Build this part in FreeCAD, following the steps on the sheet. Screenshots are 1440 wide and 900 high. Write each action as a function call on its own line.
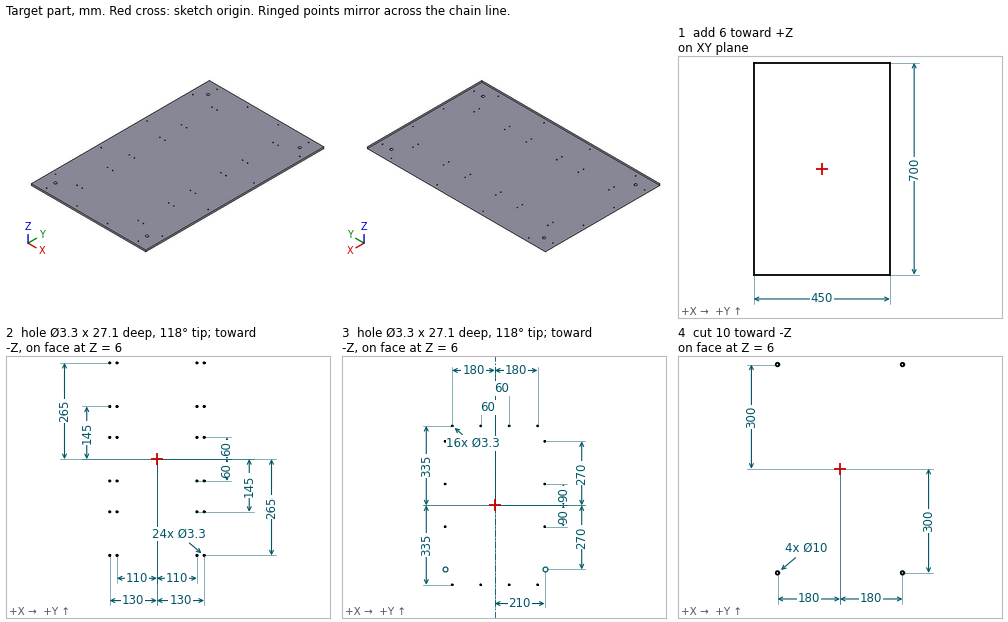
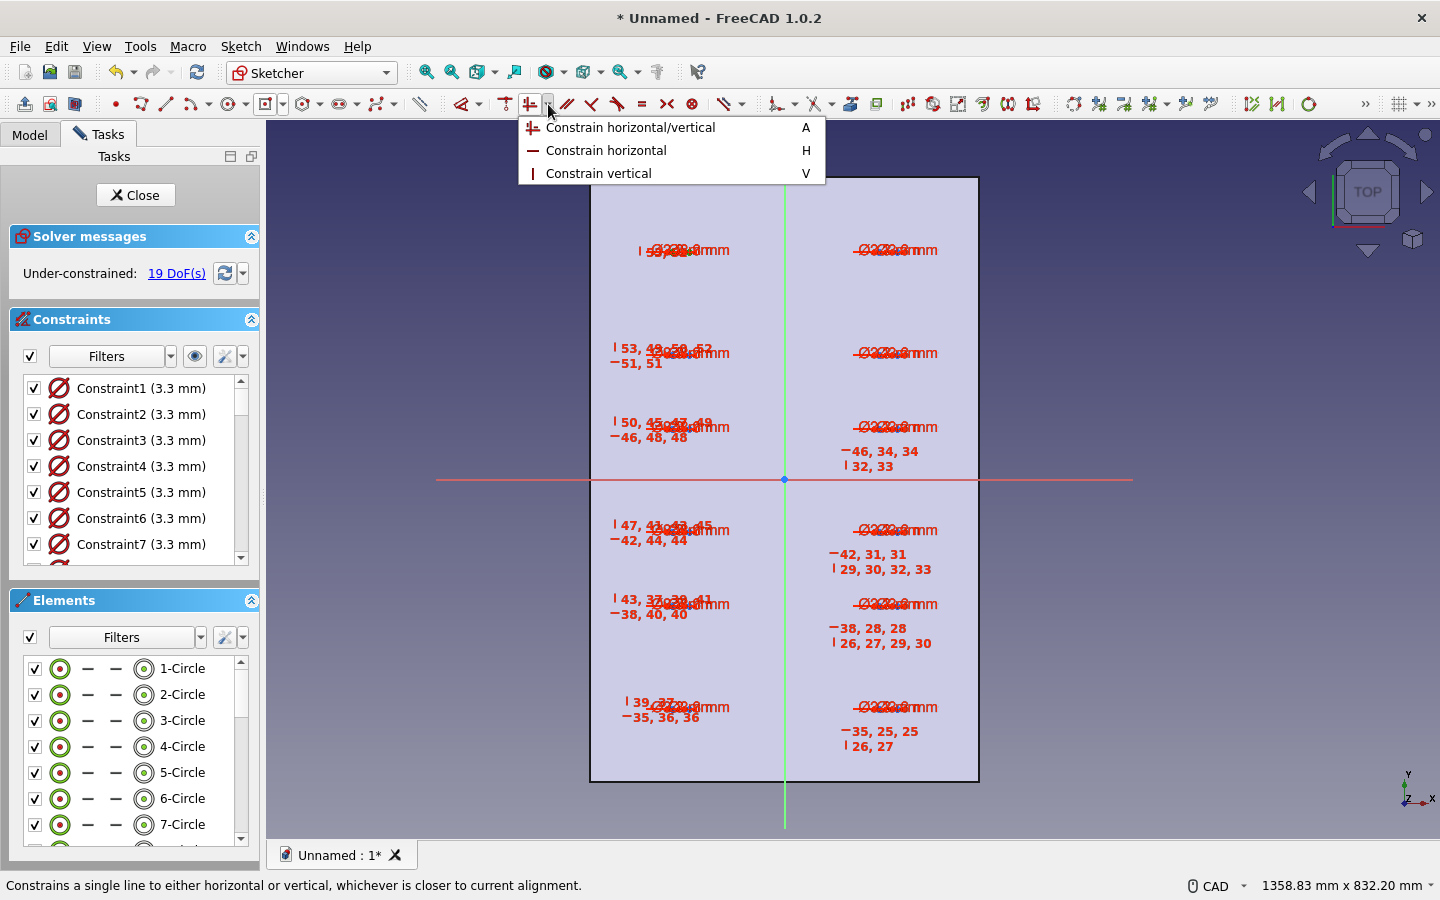
click(672, 150)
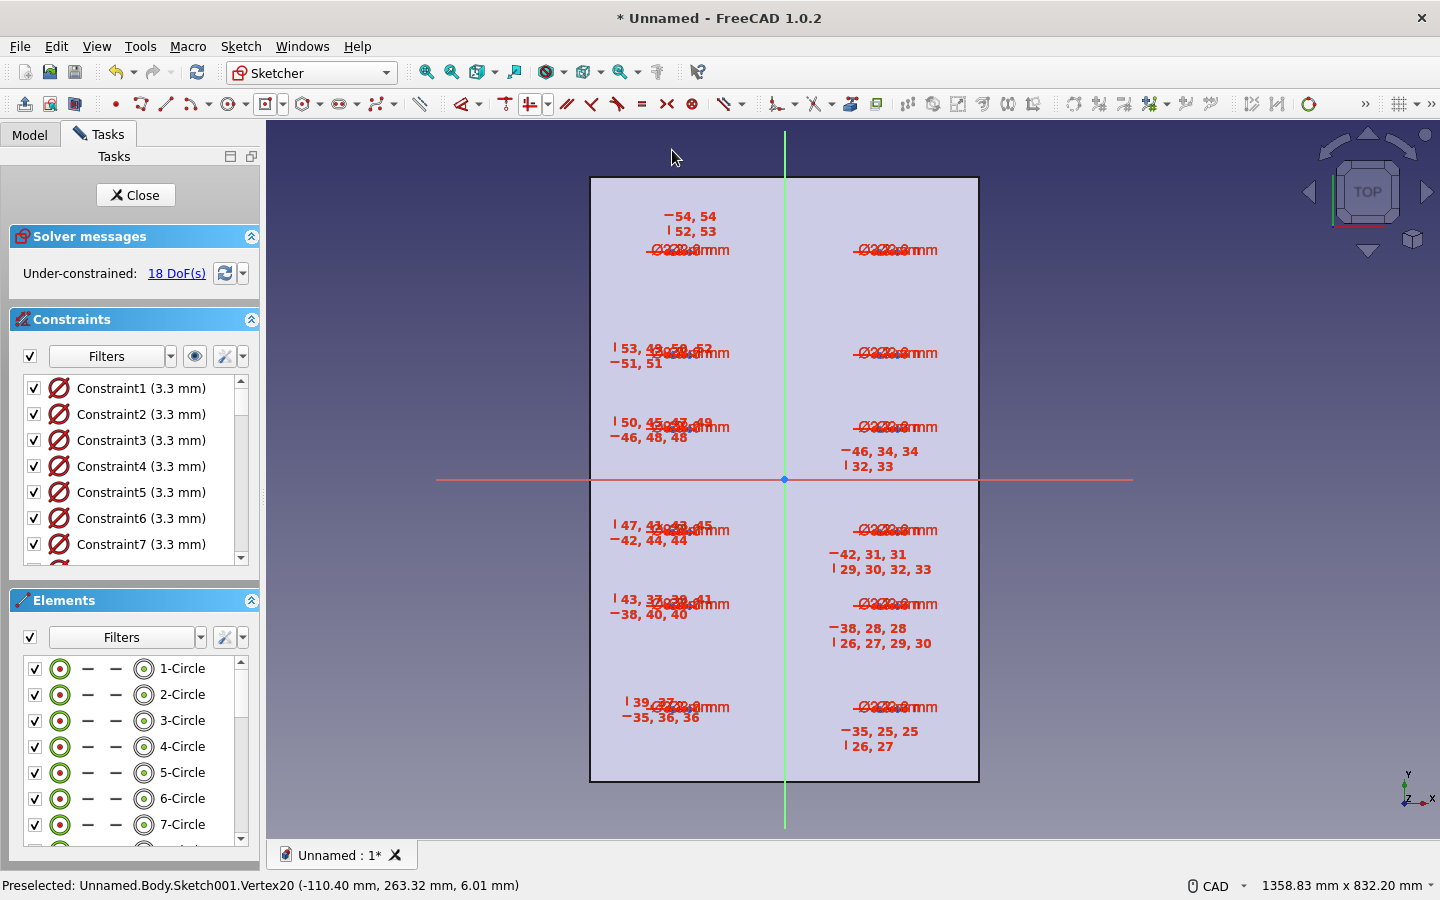
click(879, 429)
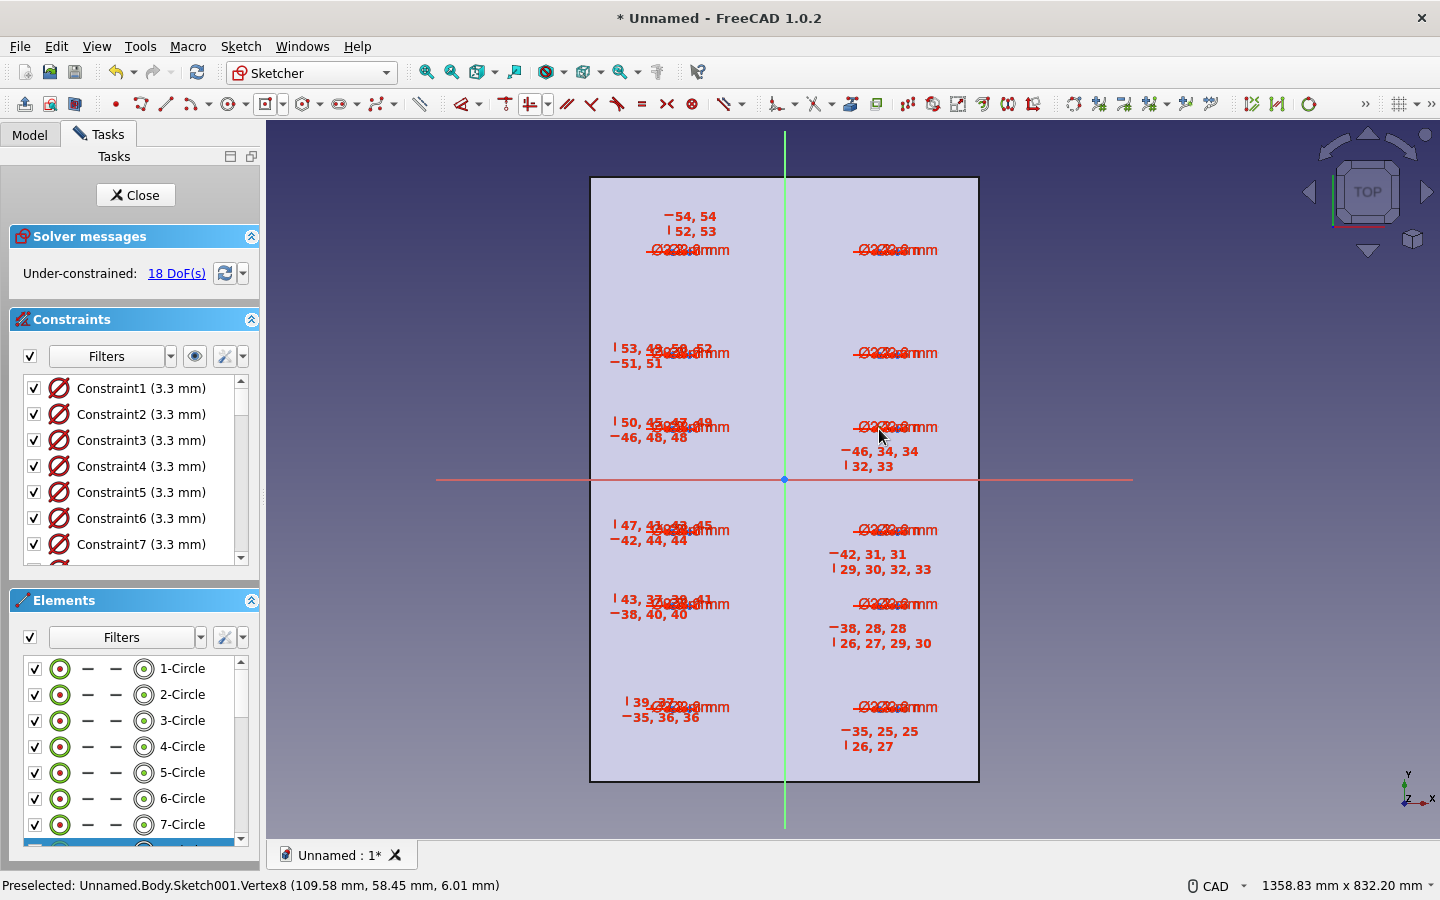
click(879, 355)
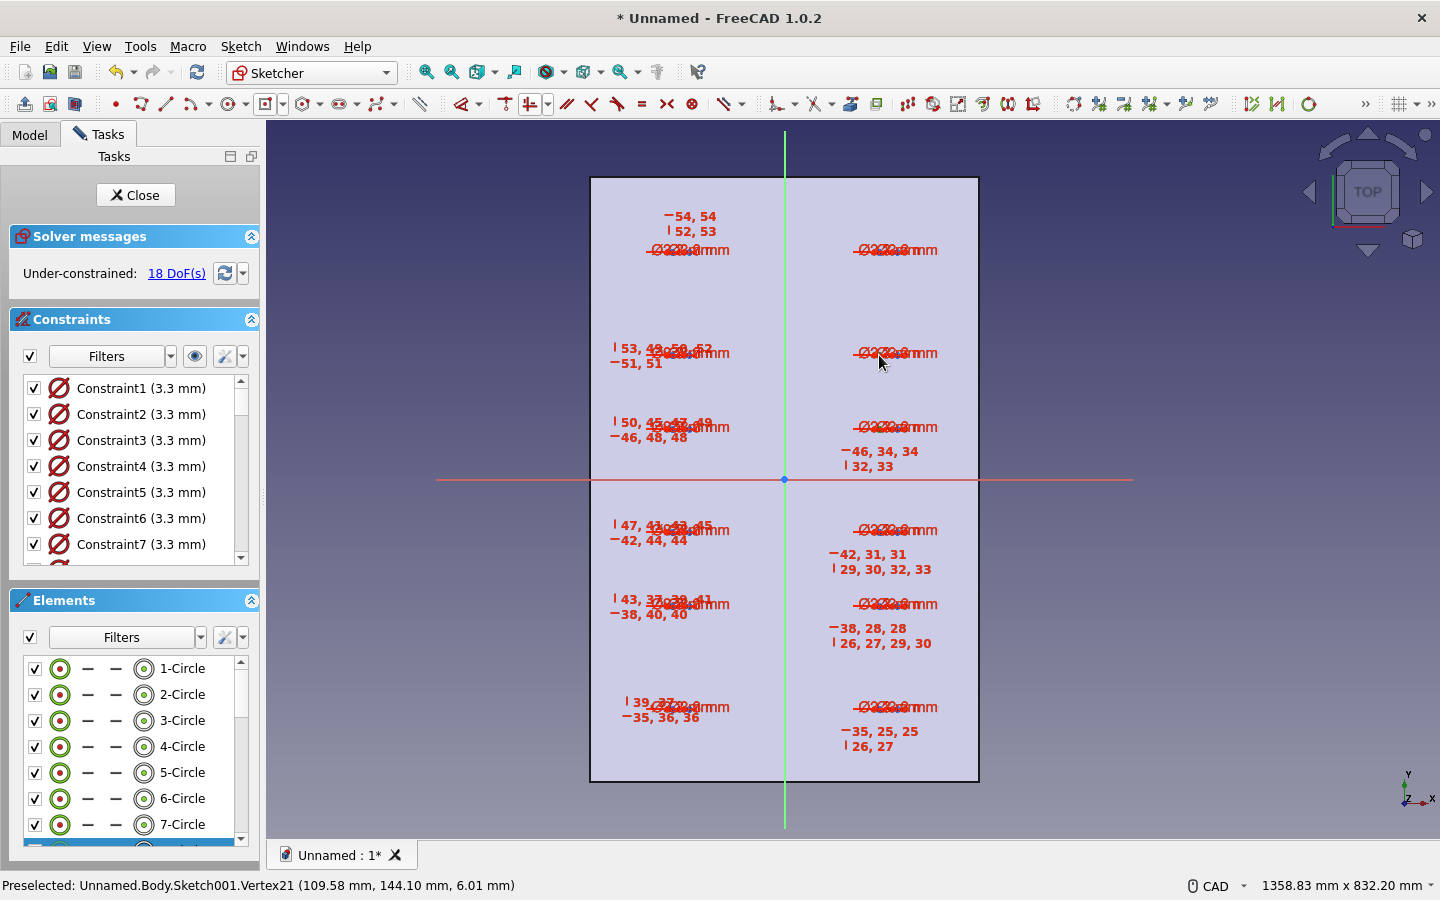
key(v)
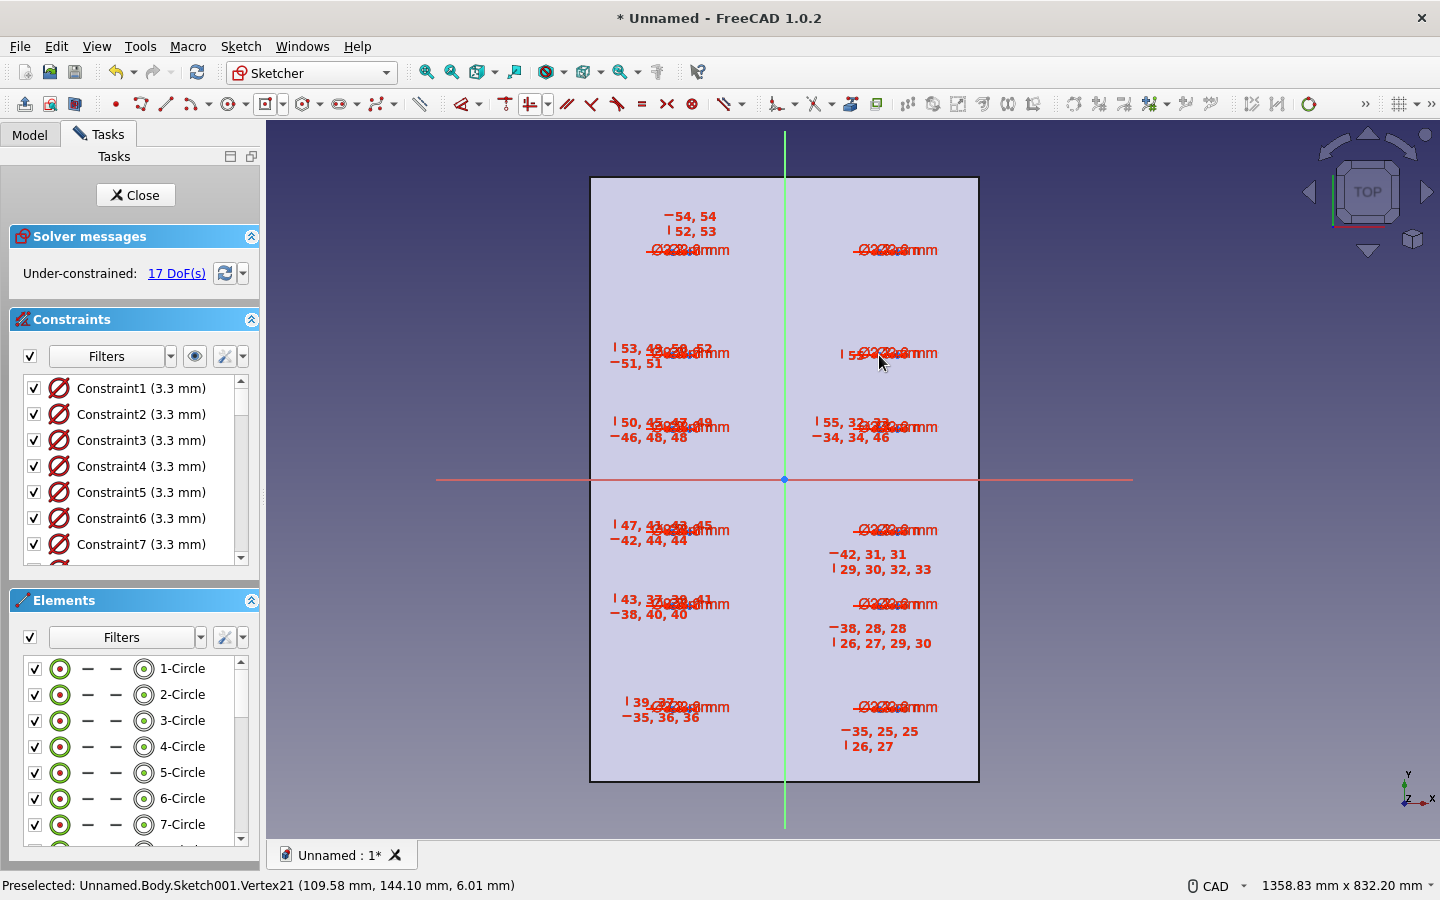
click(689, 355)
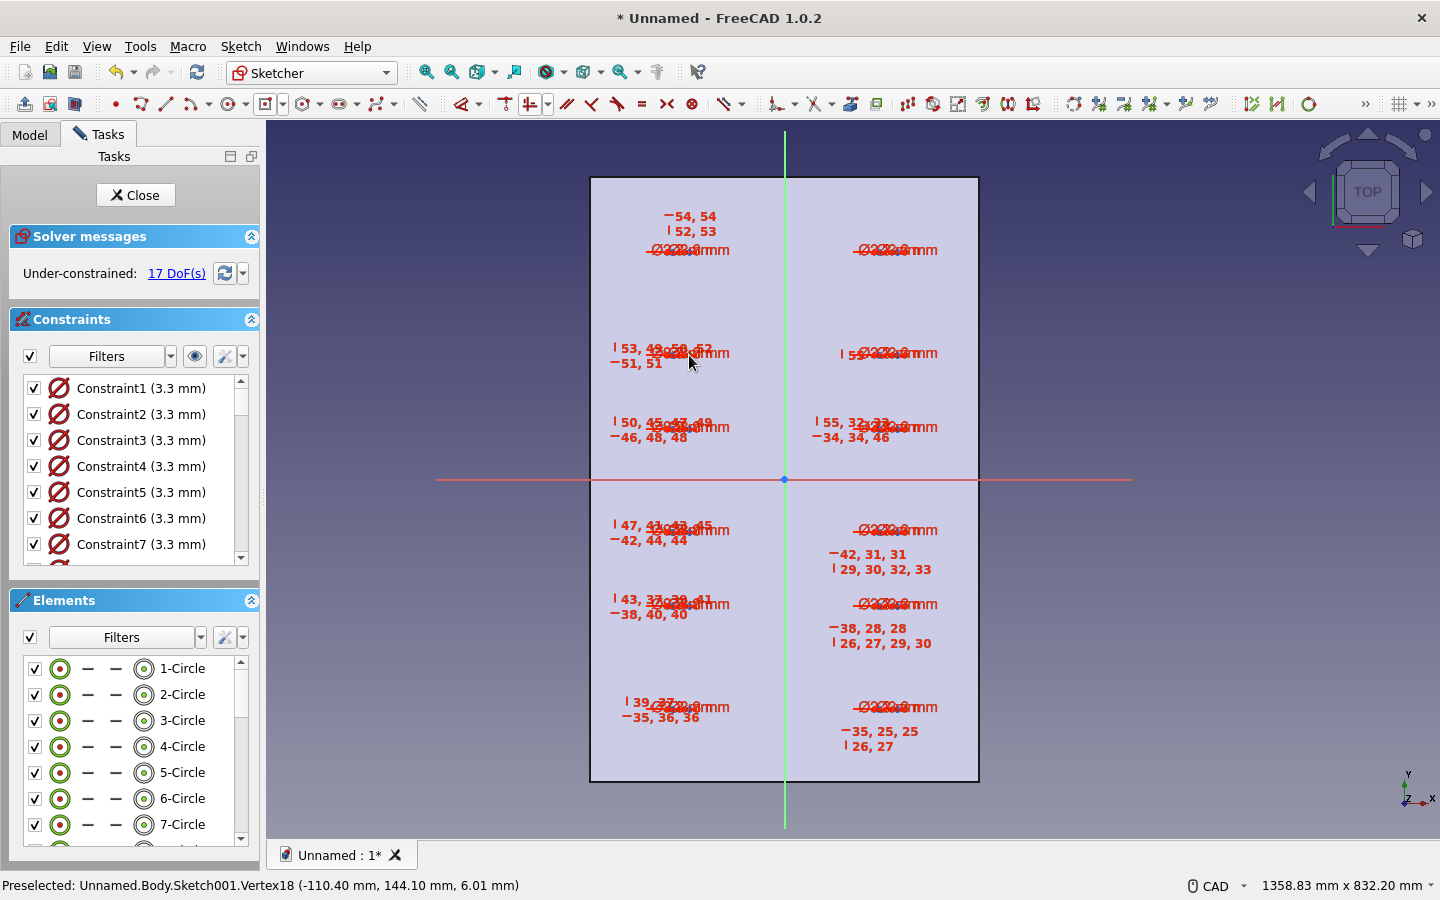
click(879, 355)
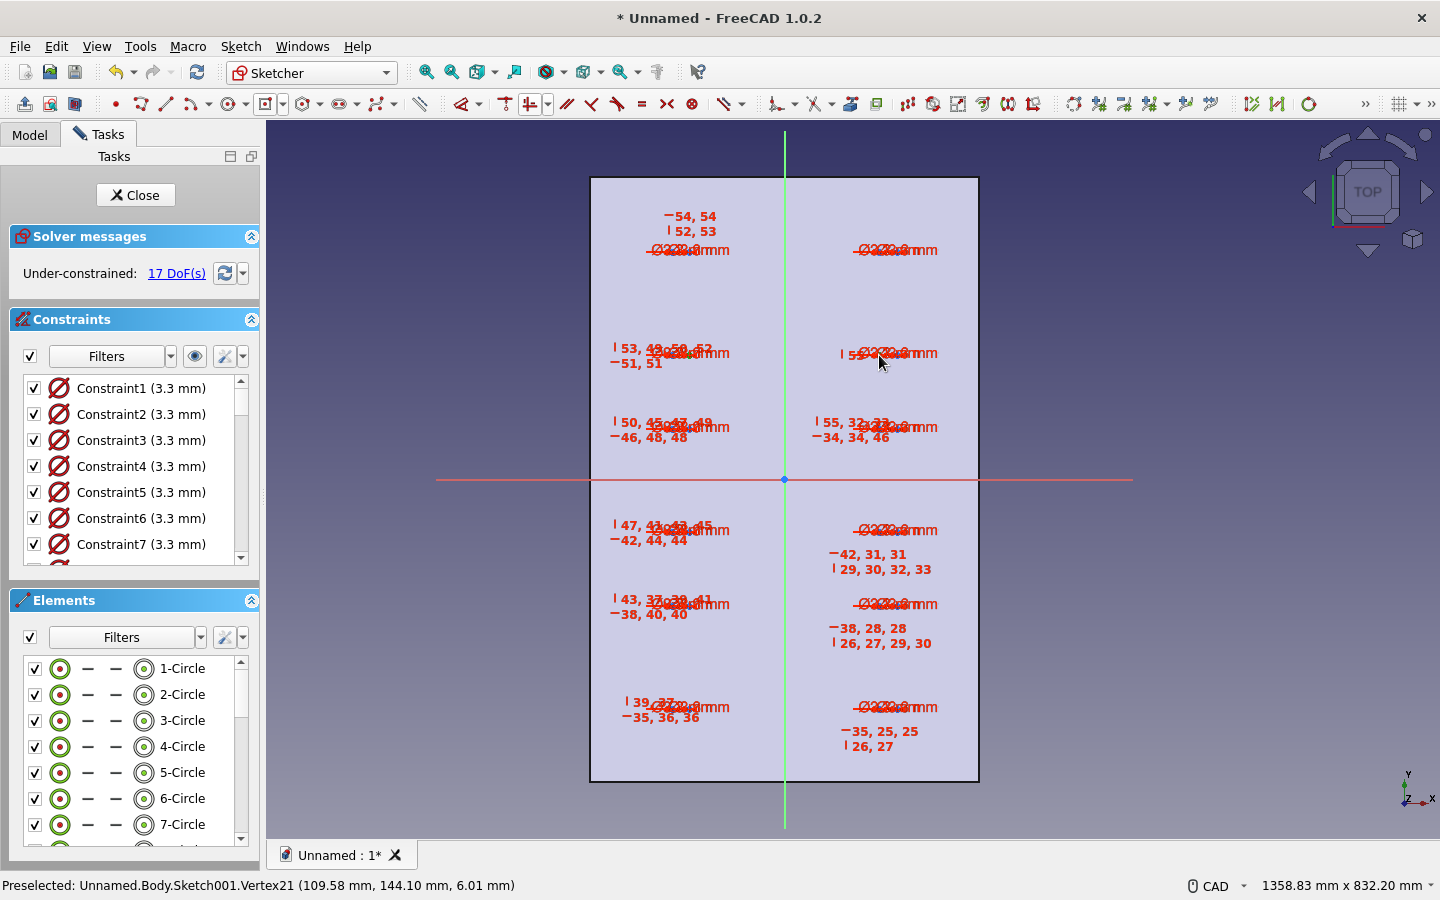
click(548, 104)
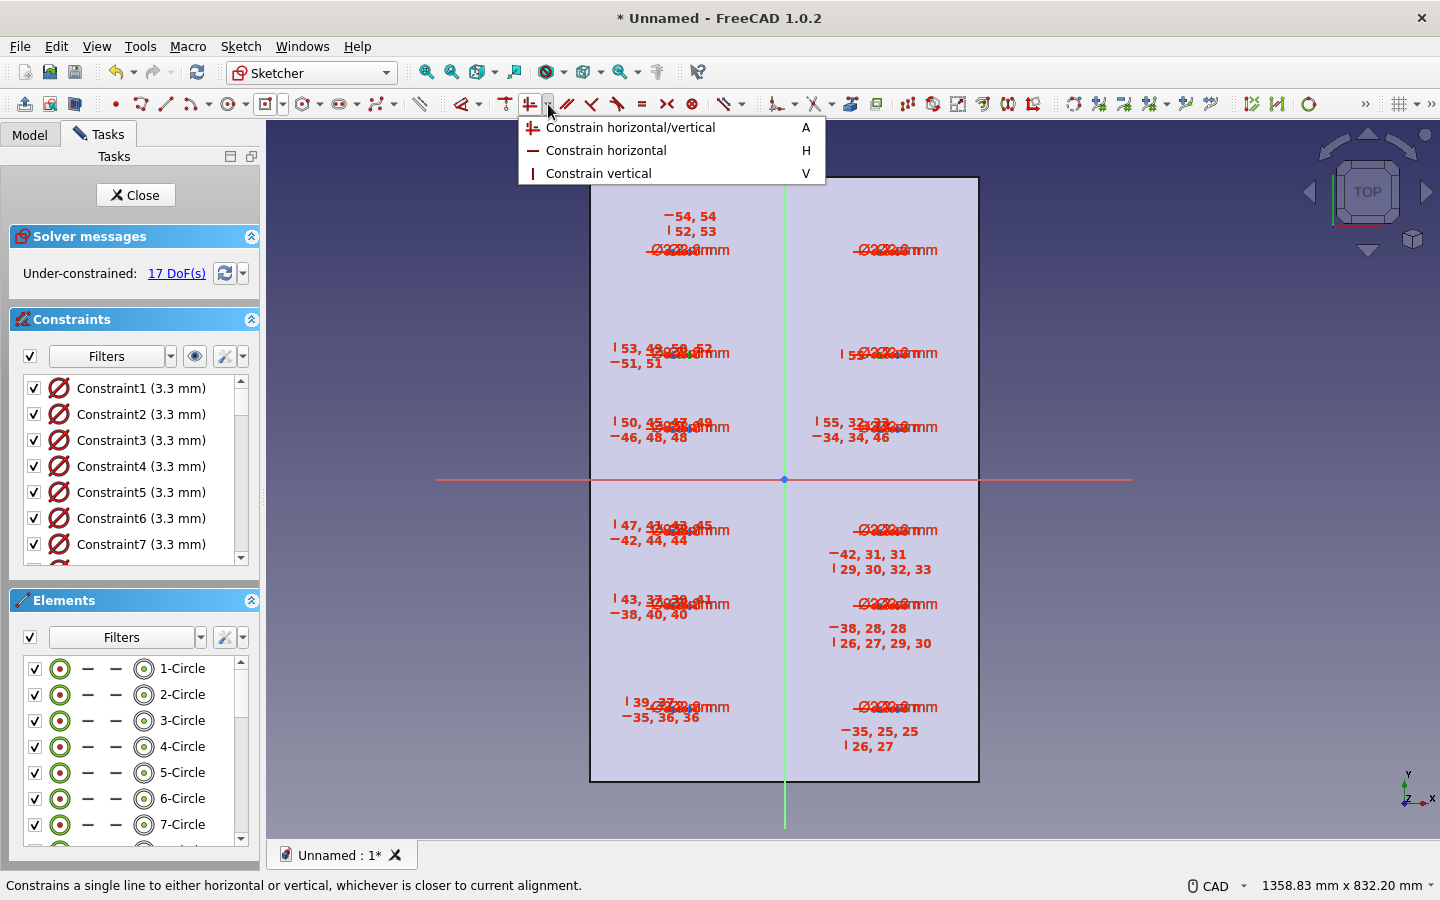
click(672, 150)